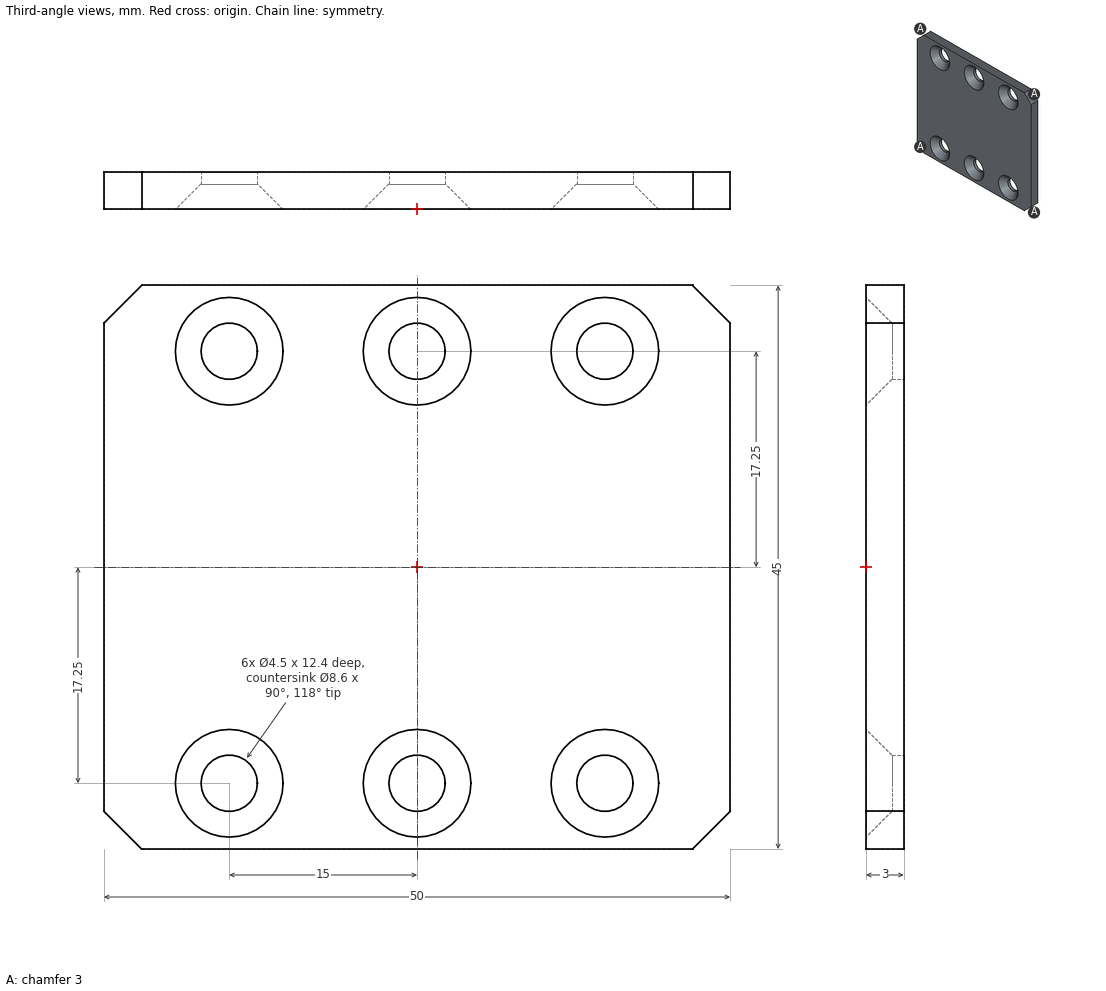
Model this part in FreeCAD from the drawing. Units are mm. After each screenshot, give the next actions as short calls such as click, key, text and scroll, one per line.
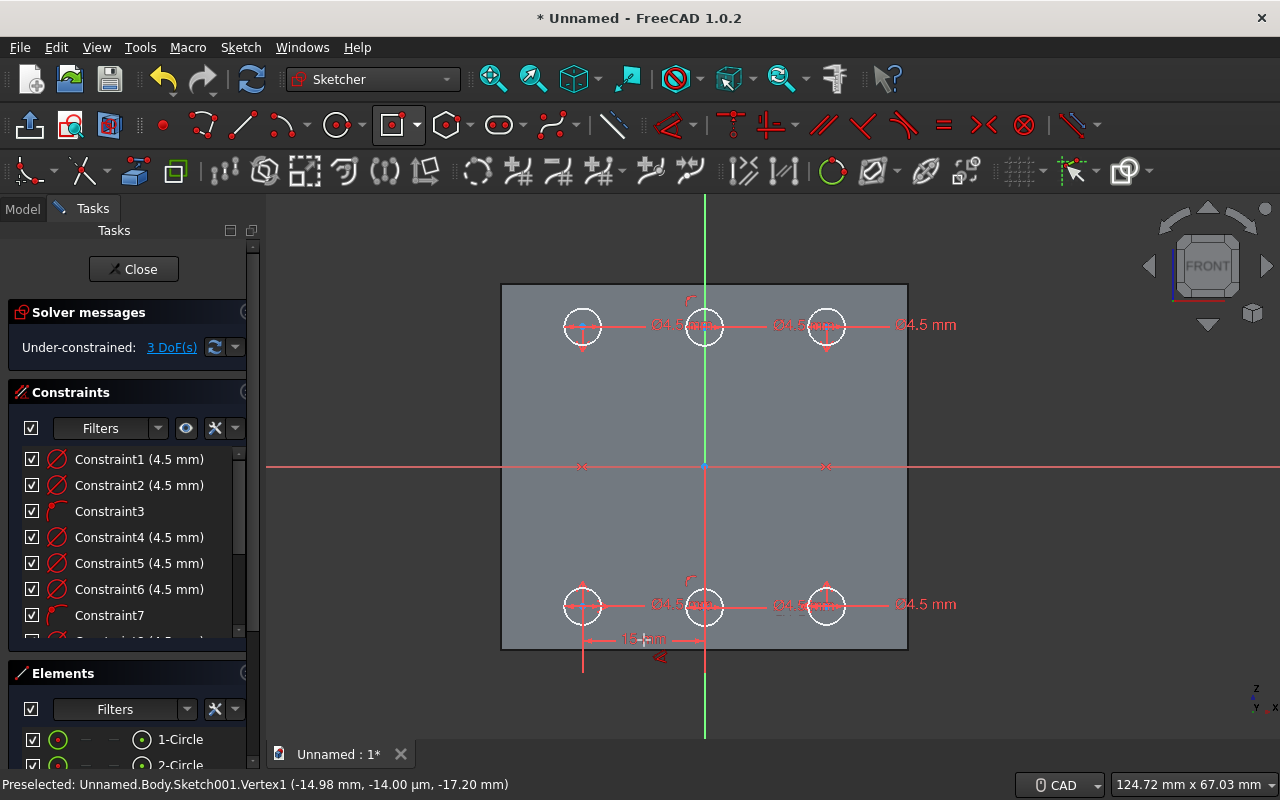
click(583, 606)
click(549, 537)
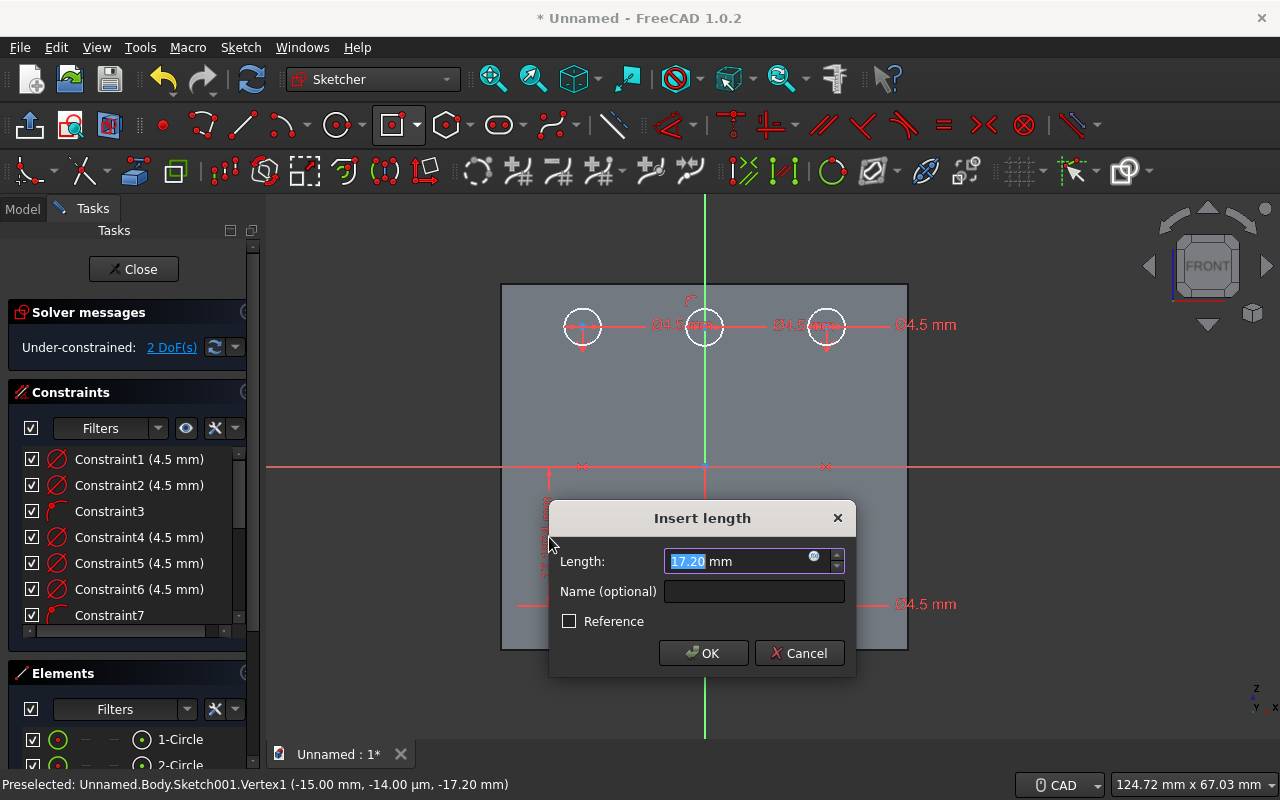
text(17.25)
key(Return)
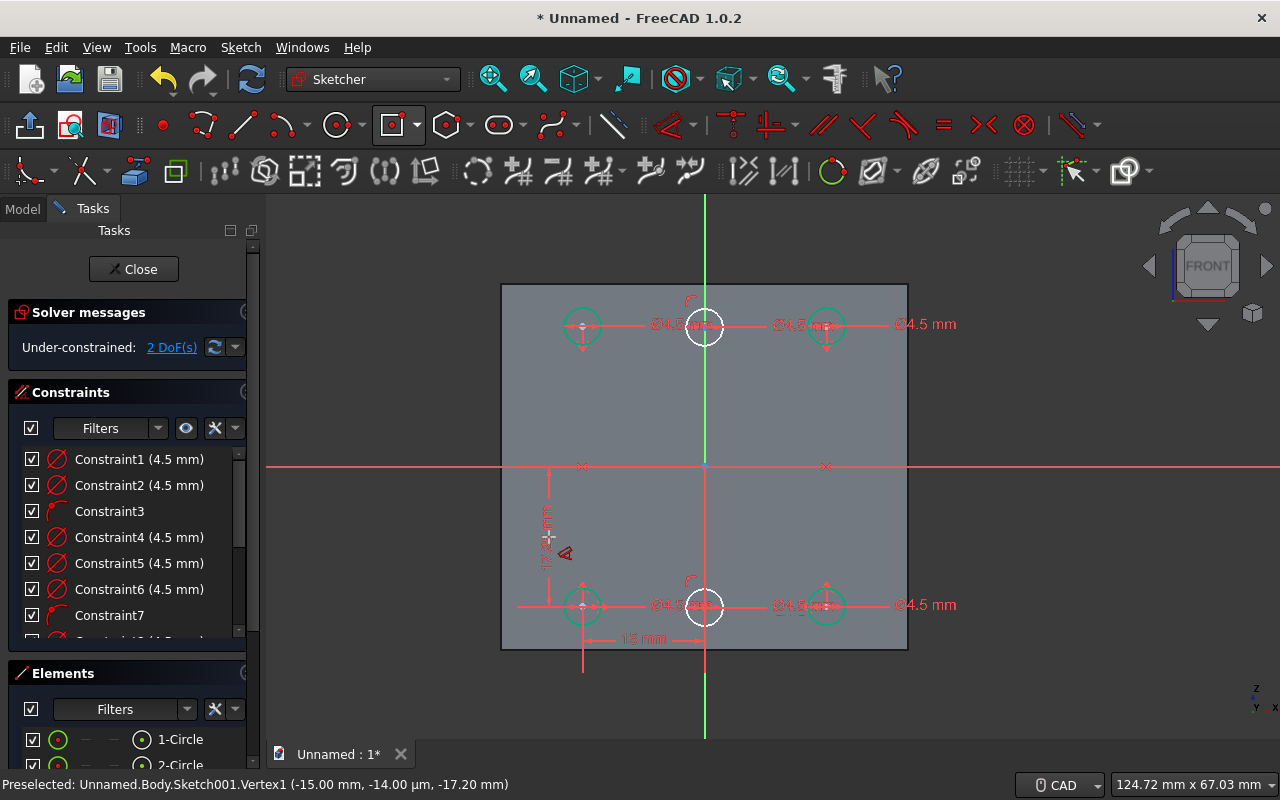
click(705, 608)
click(739, 537)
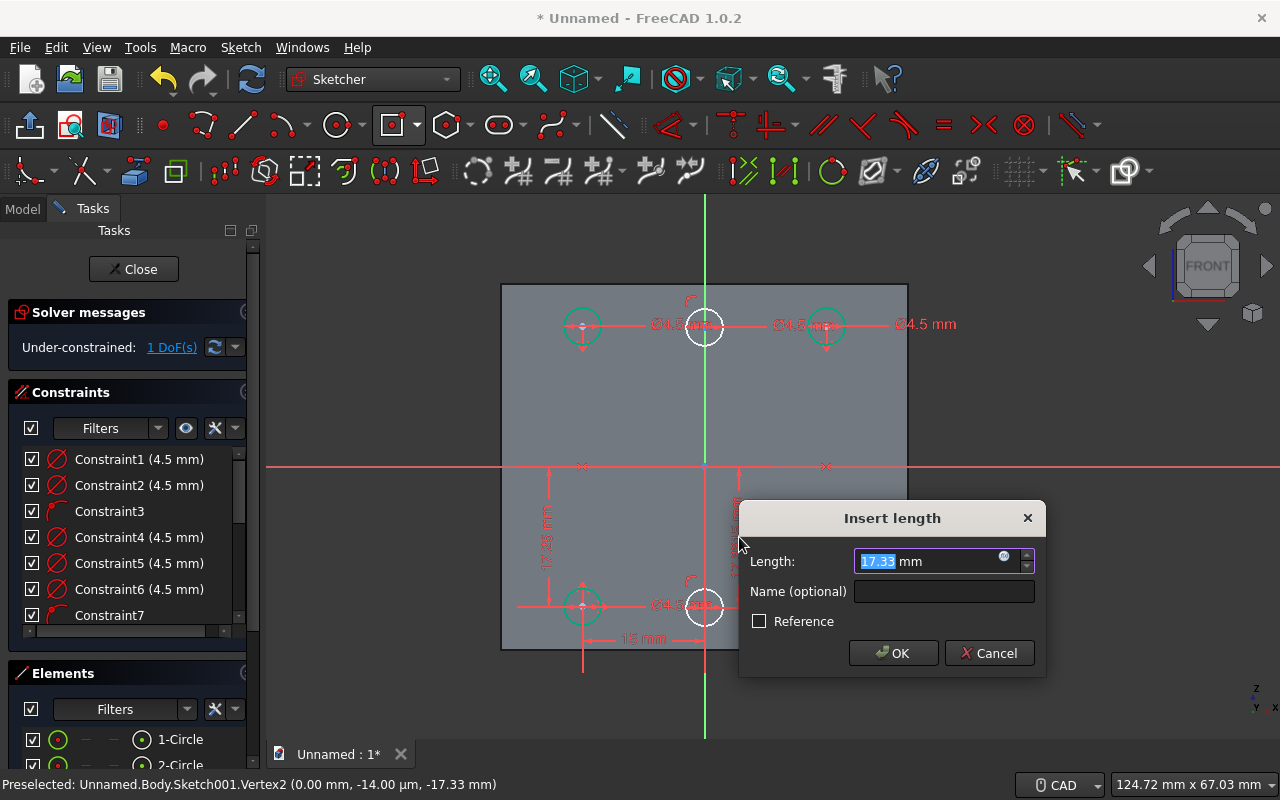
text(17.25)
key(Return)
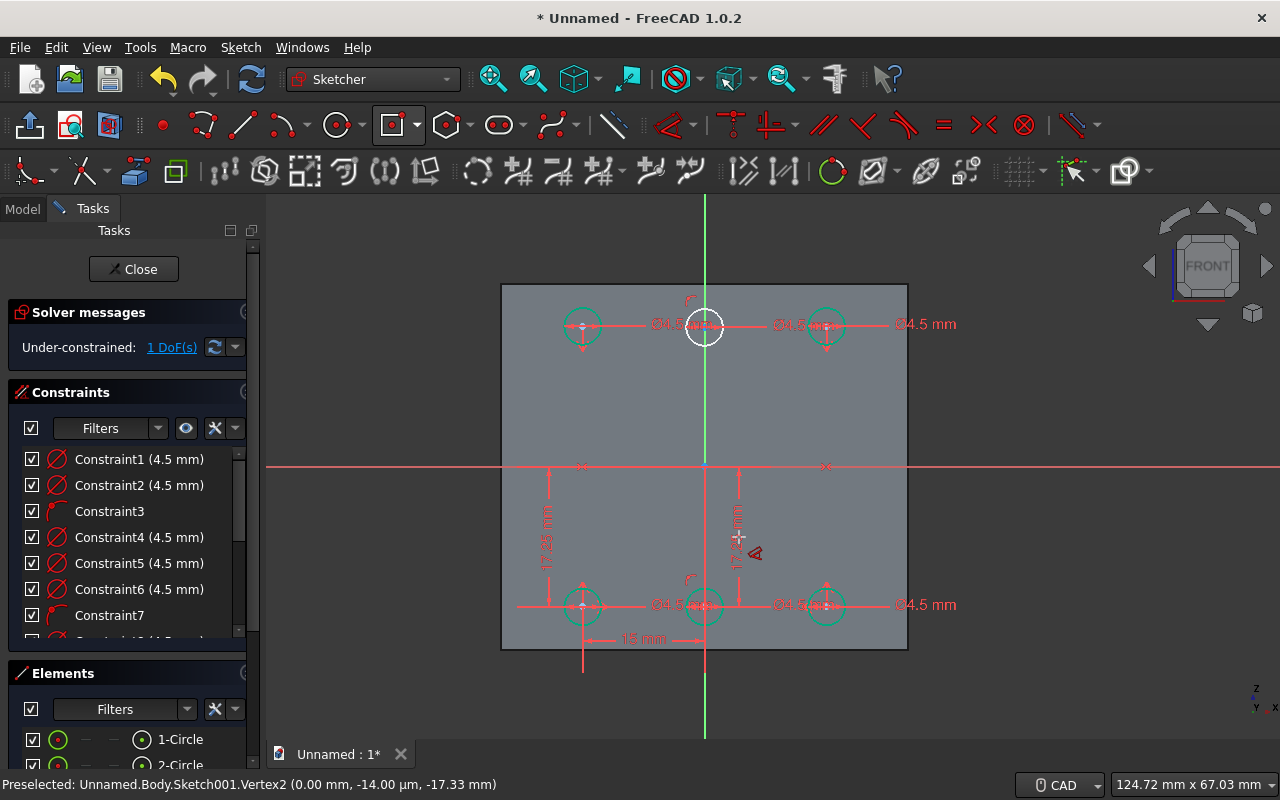
click(705, 327)
click(739, 397)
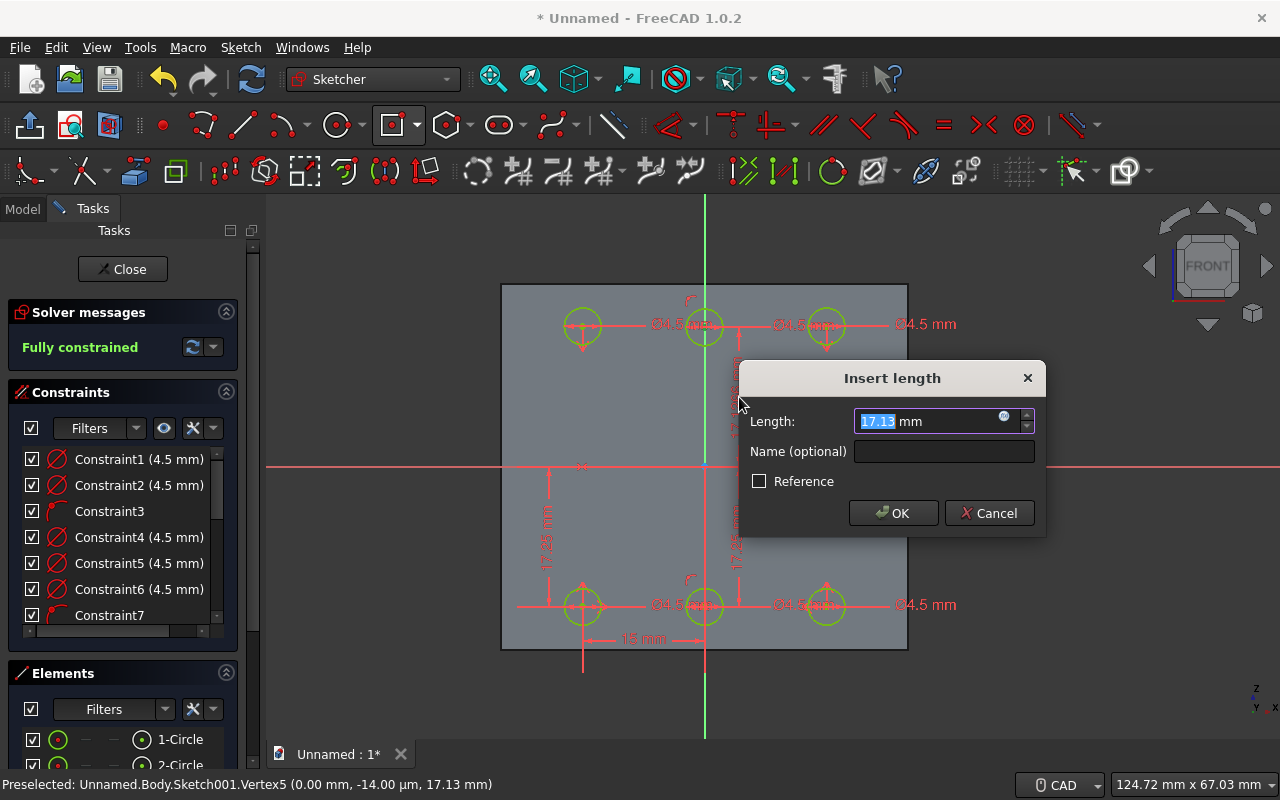
text(17.25)
key(Return)
key(Escape)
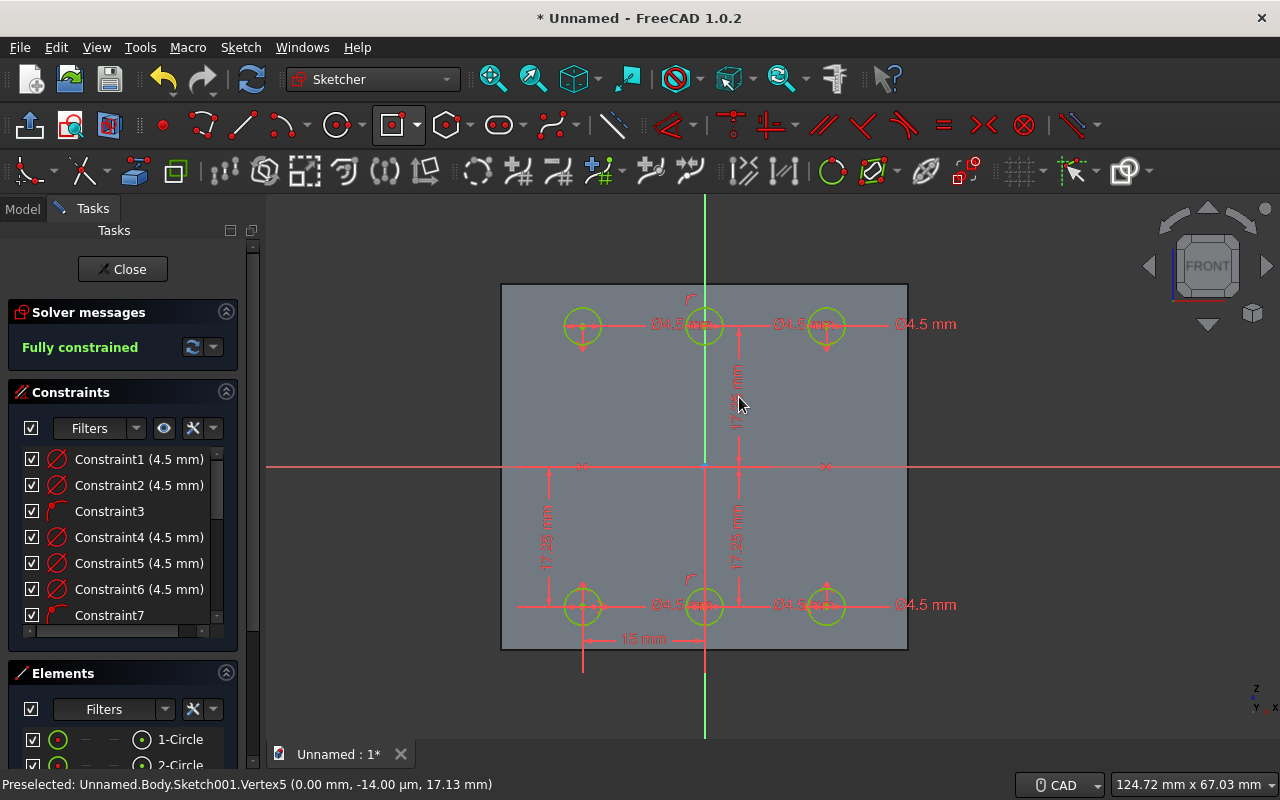
click(123, 269)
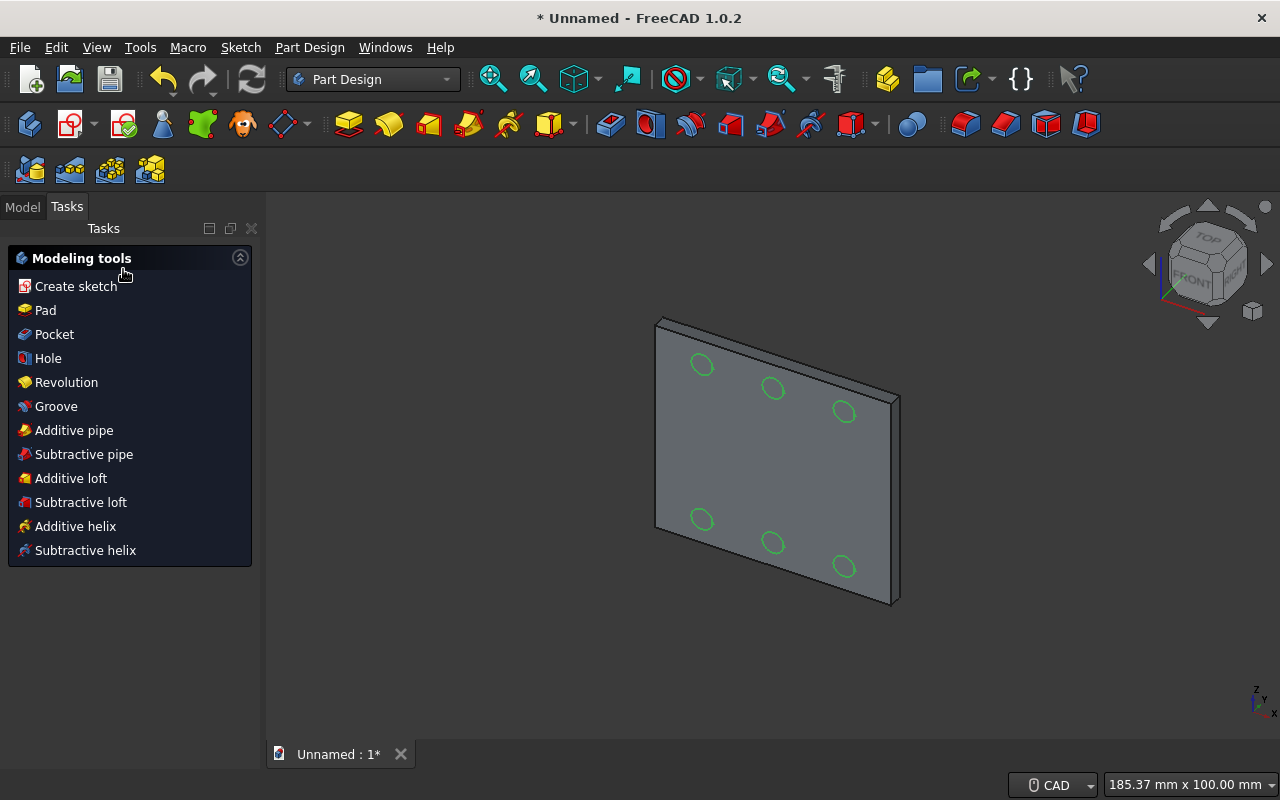
click(652, 124)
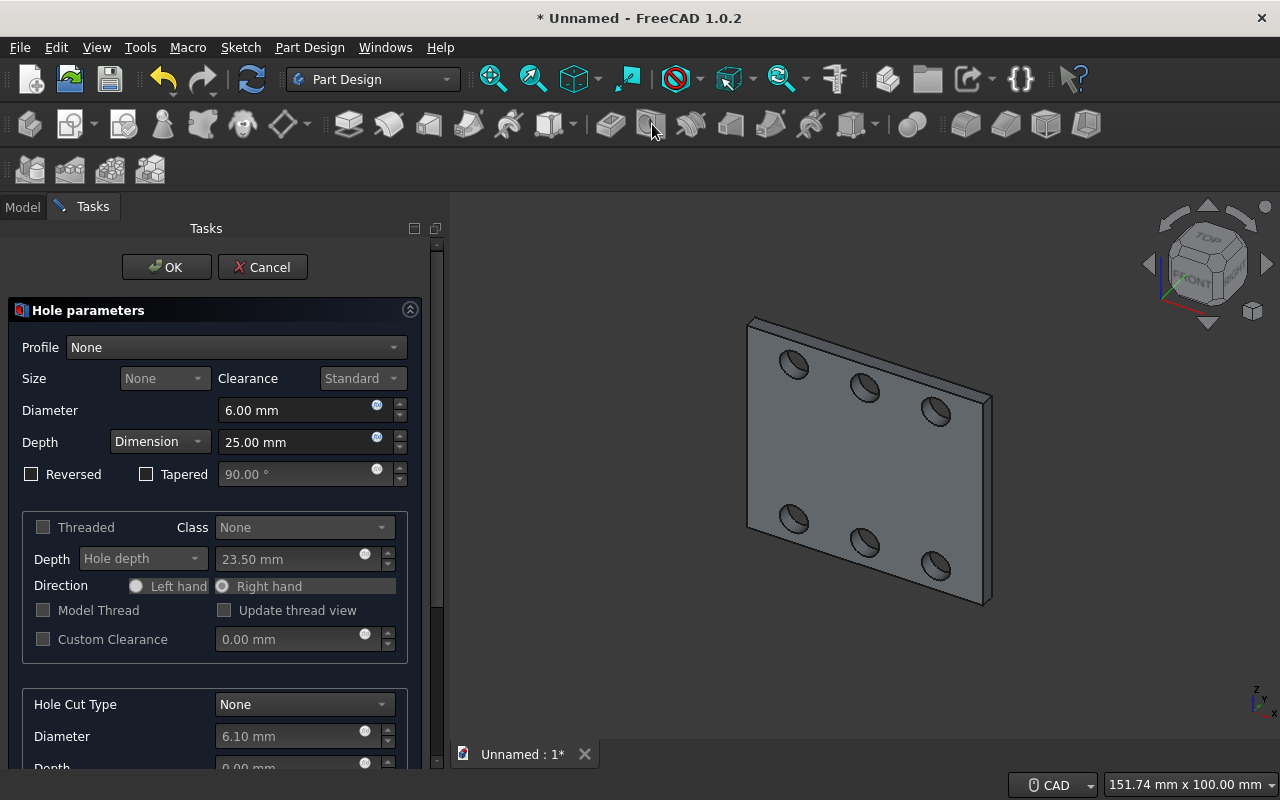
triple_click(305, 410)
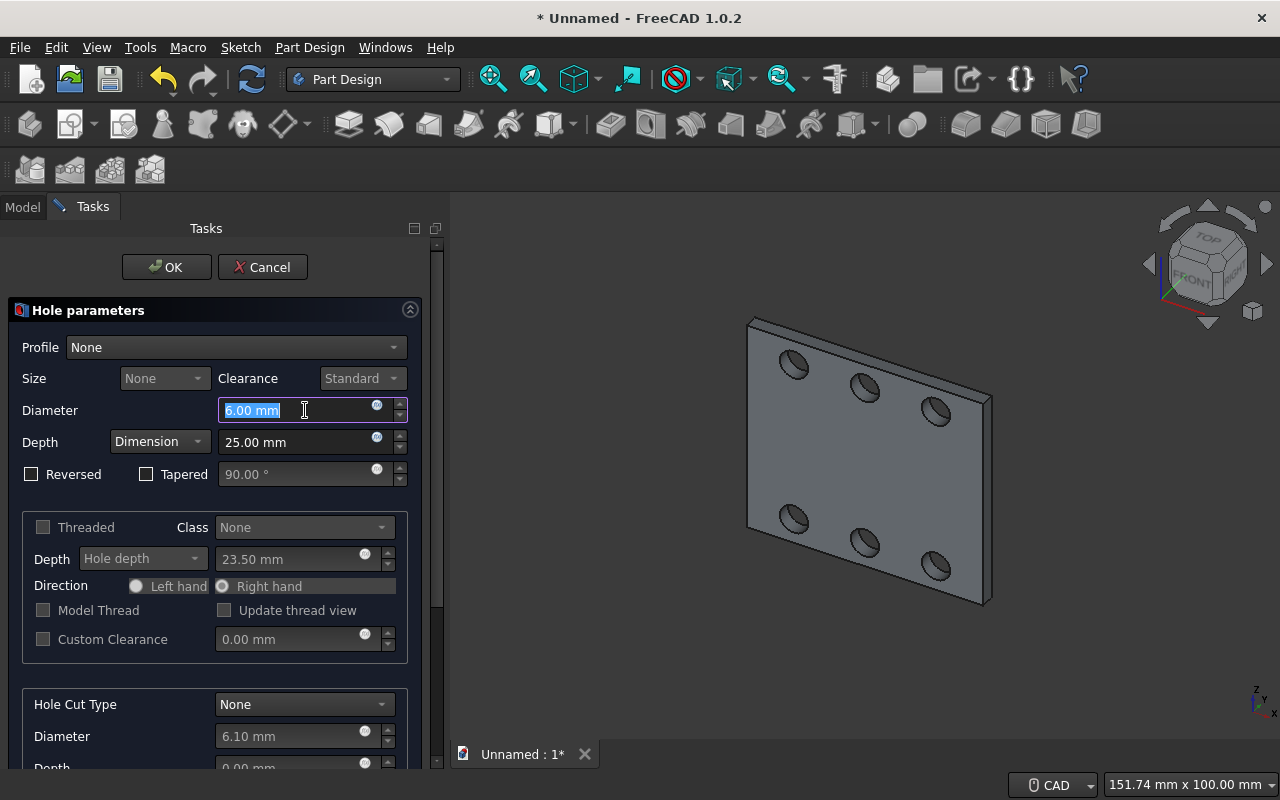
text(4.5)
key(Tab)